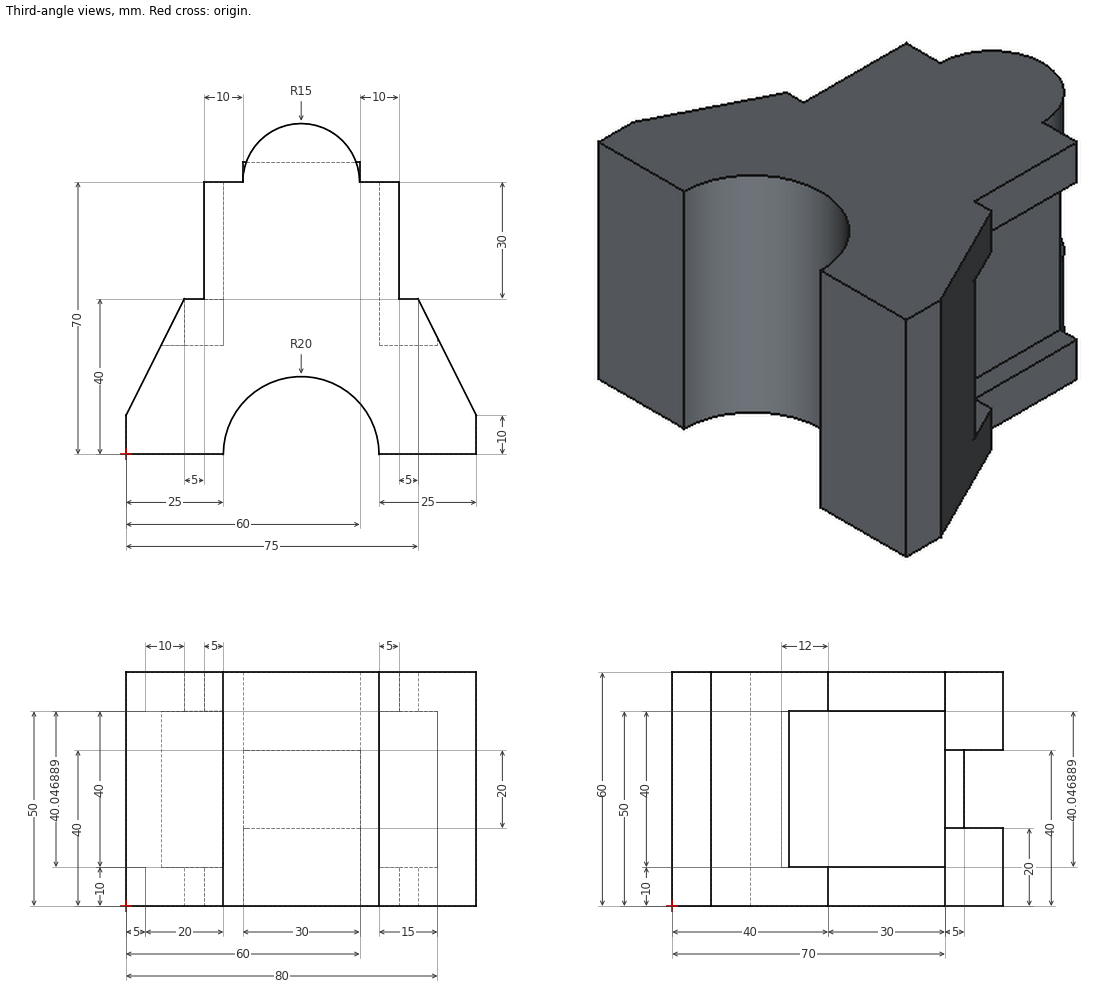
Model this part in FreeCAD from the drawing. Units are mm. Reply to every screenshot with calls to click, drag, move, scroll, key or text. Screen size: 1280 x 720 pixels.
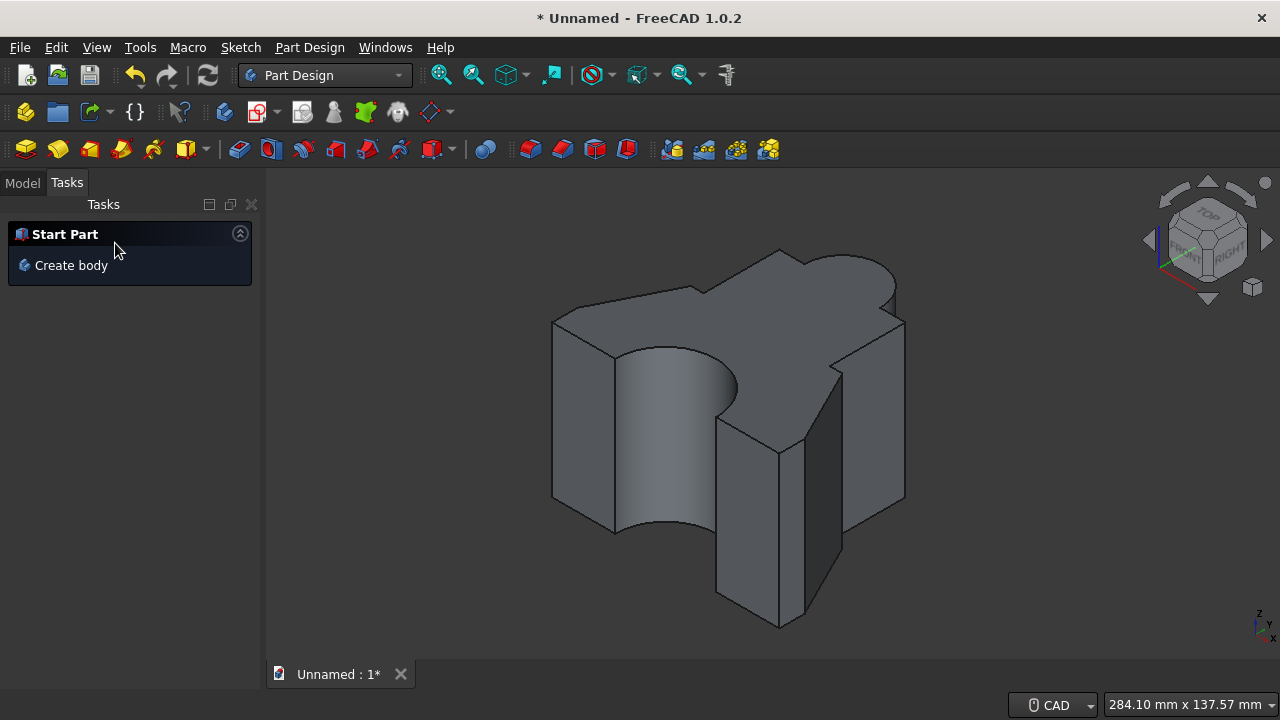
click(868, 406)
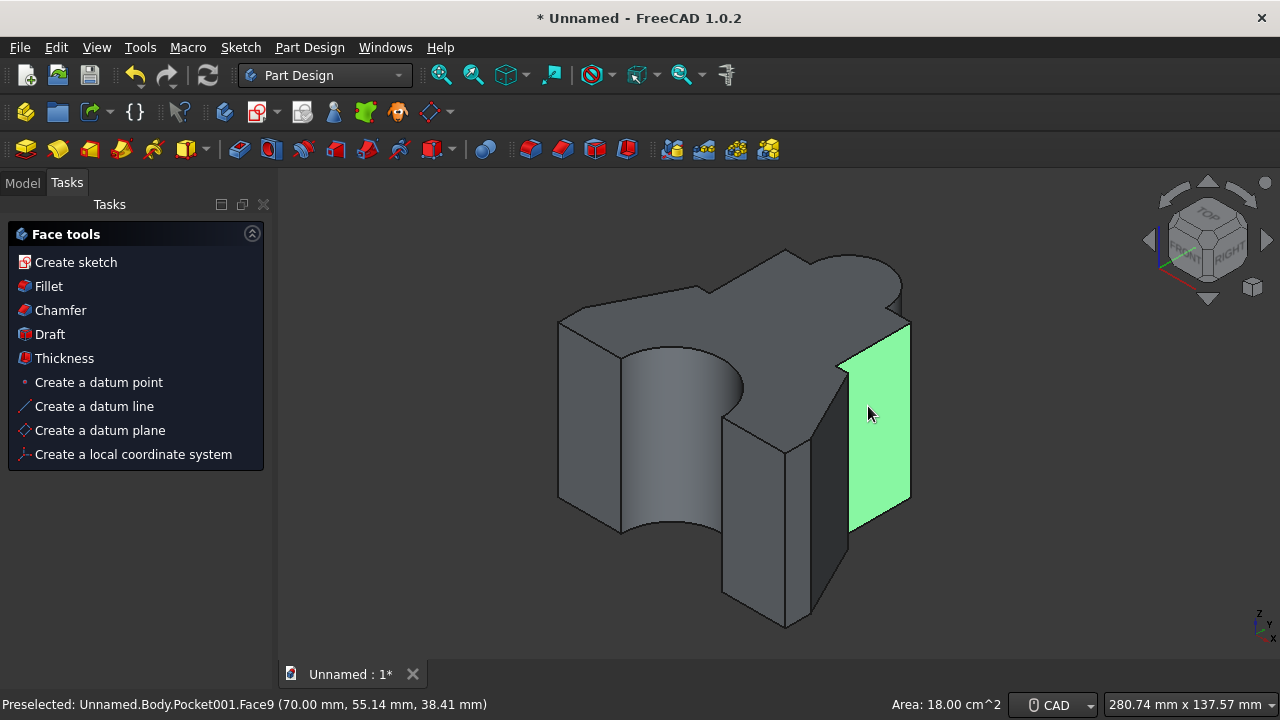
click(258, 112)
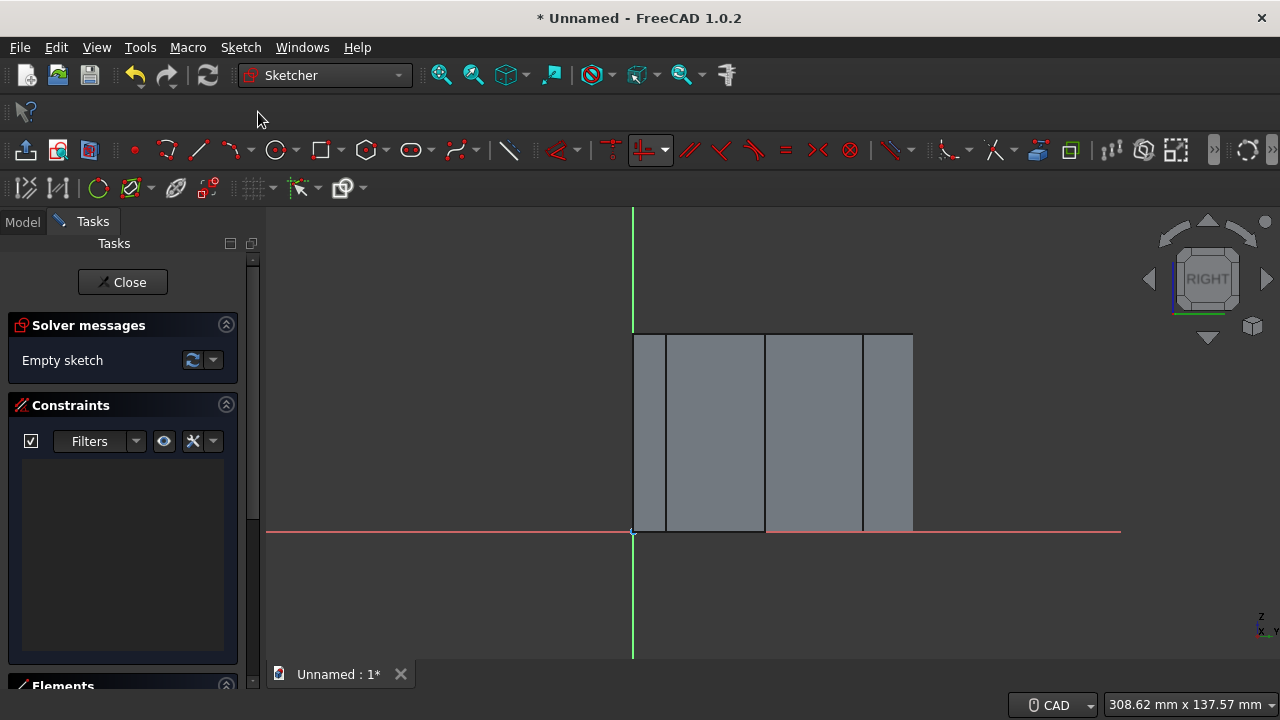
key(q)
key(s)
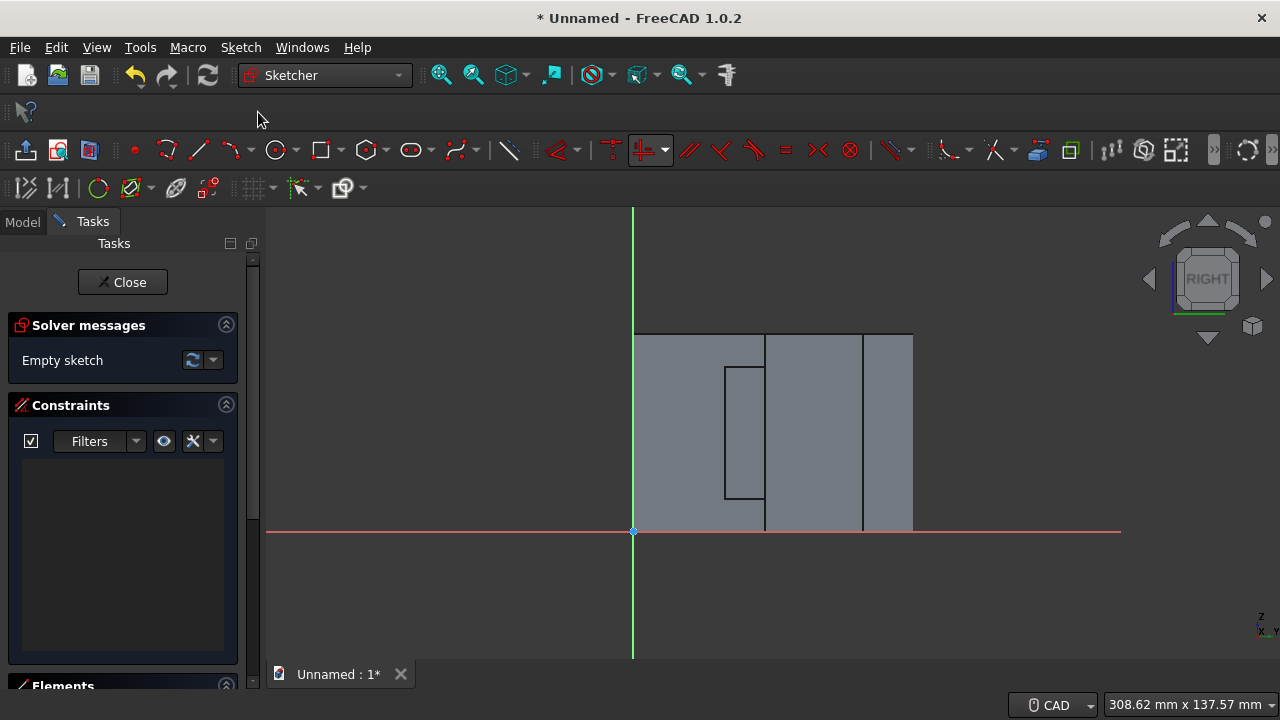
scroll(802, 469, up, 3)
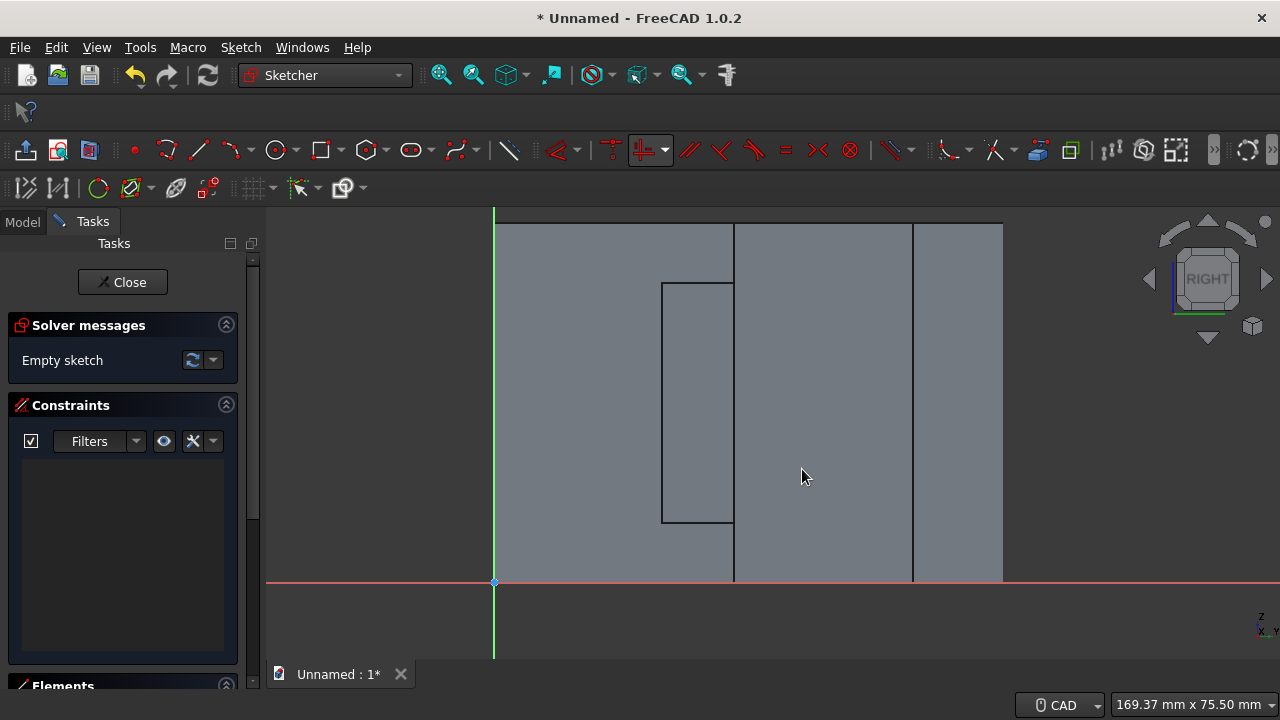
key(g)
key(r)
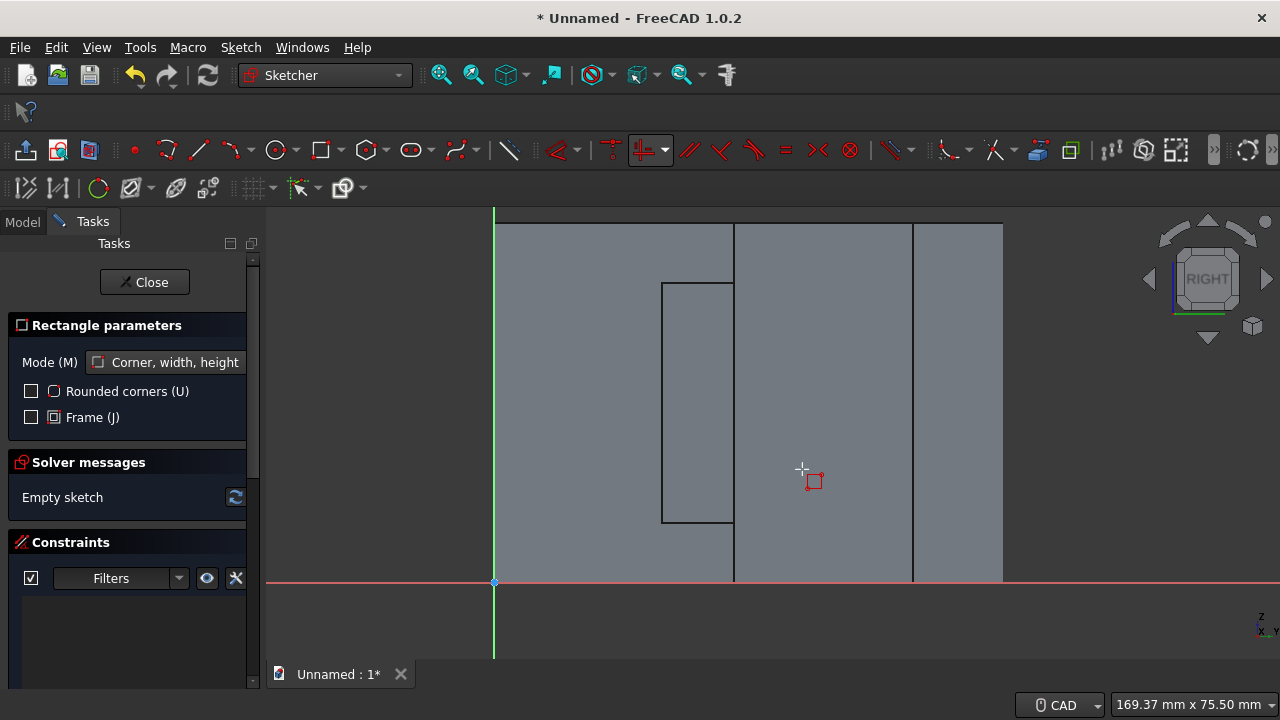
click(734, 283)
click(913, 523)
key(Escape)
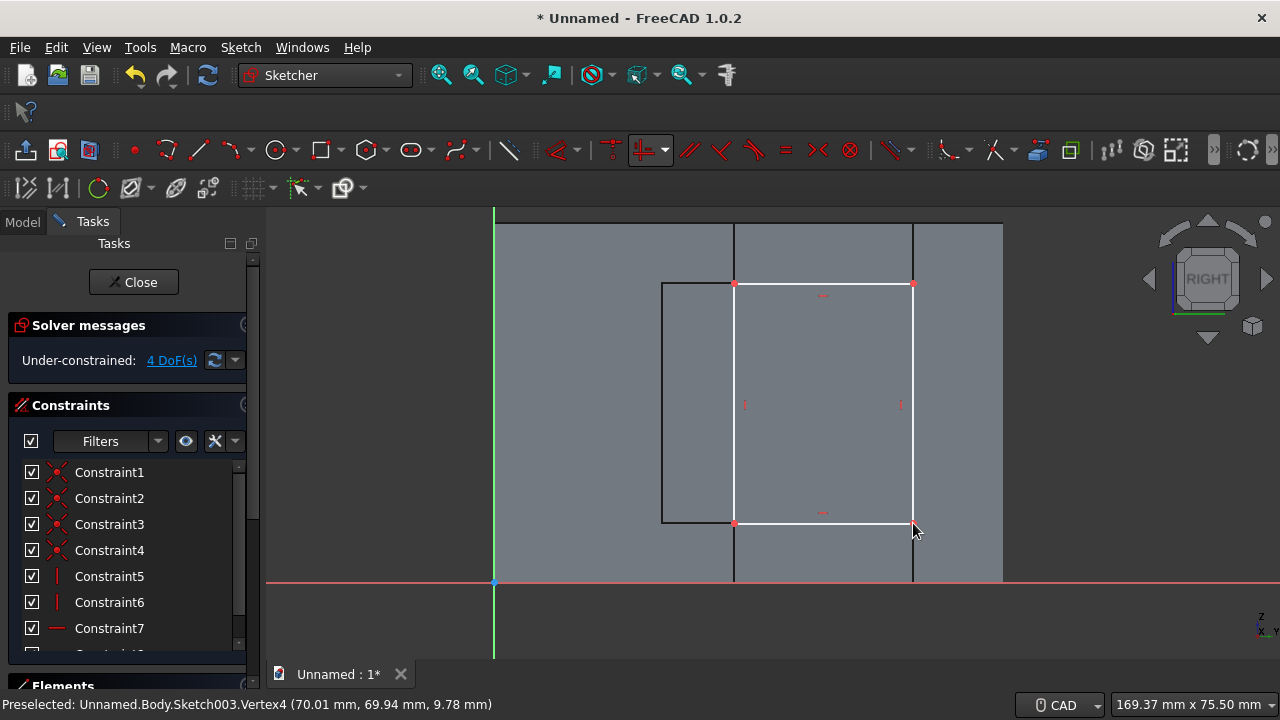
key(d)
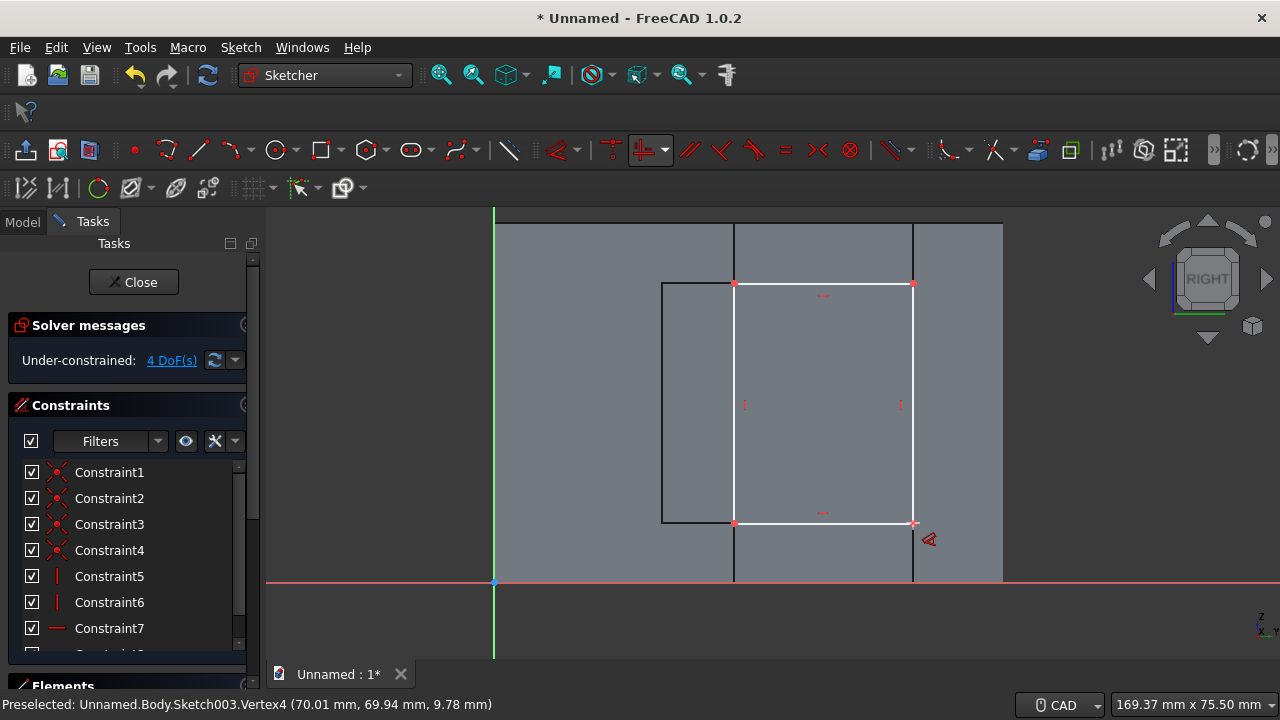
click(734, 356)
click(768, 404)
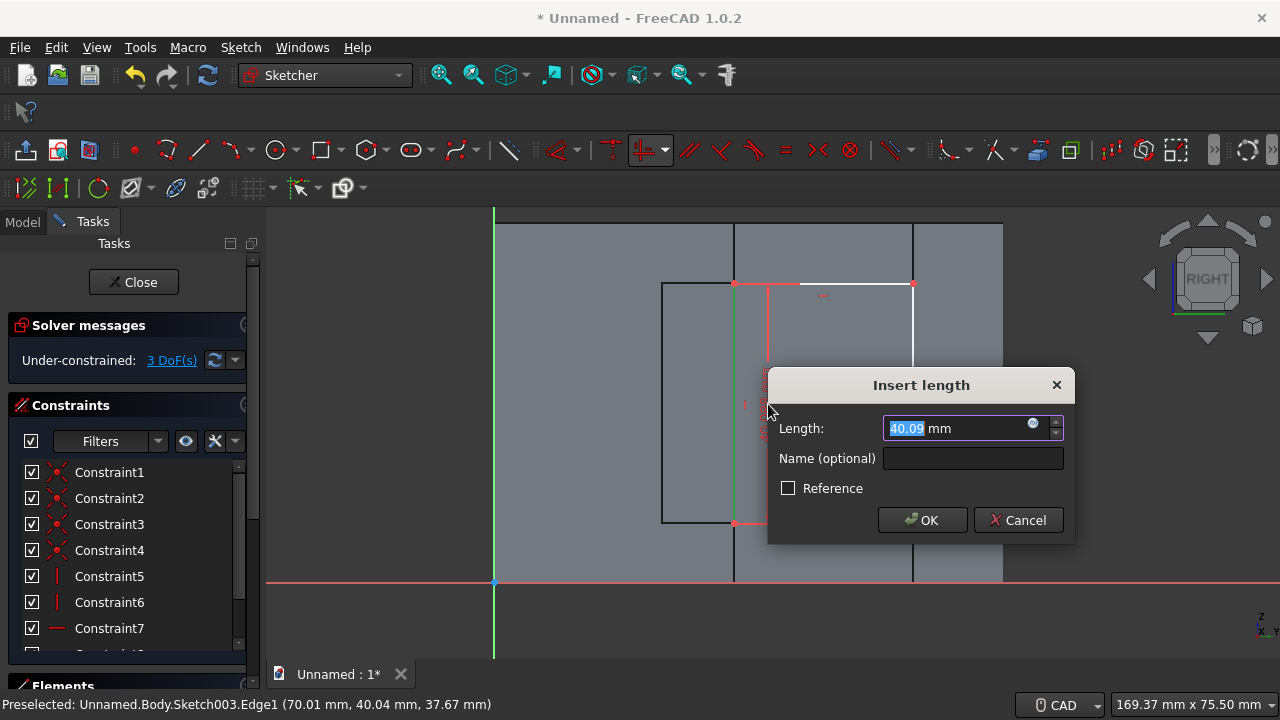
text(40)
key(Return)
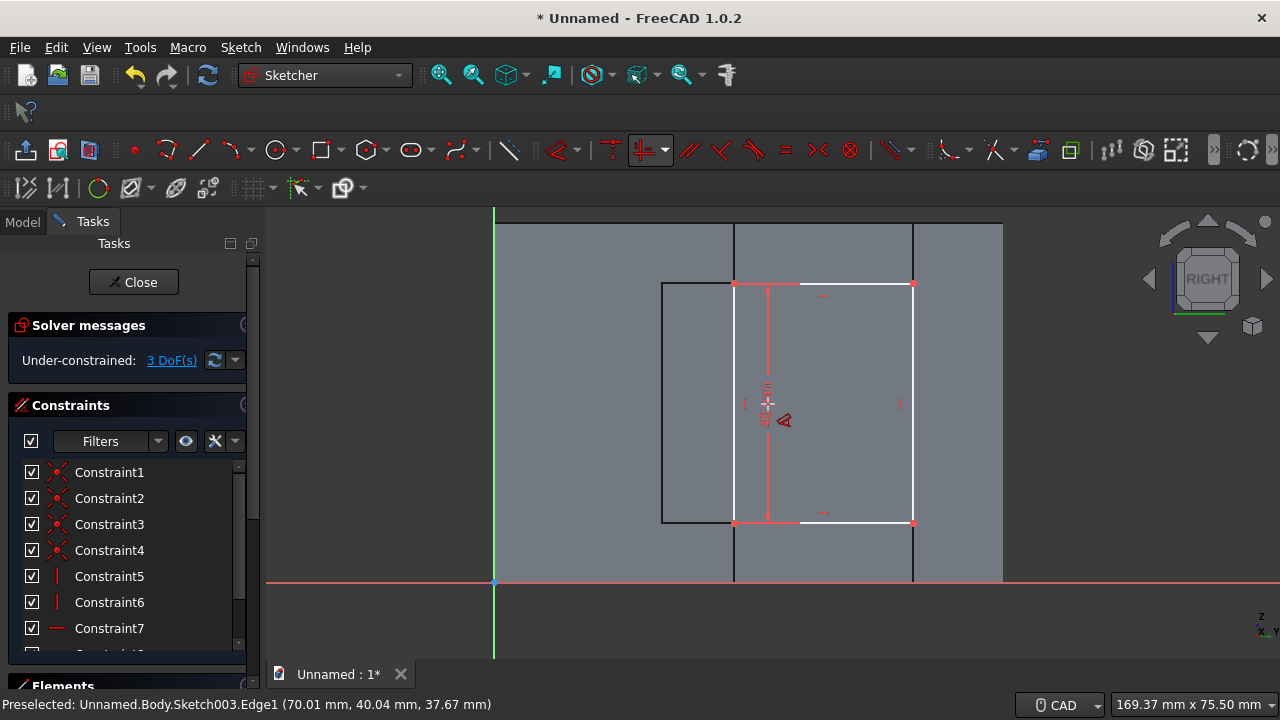
click(788, 523)
click(824, 557)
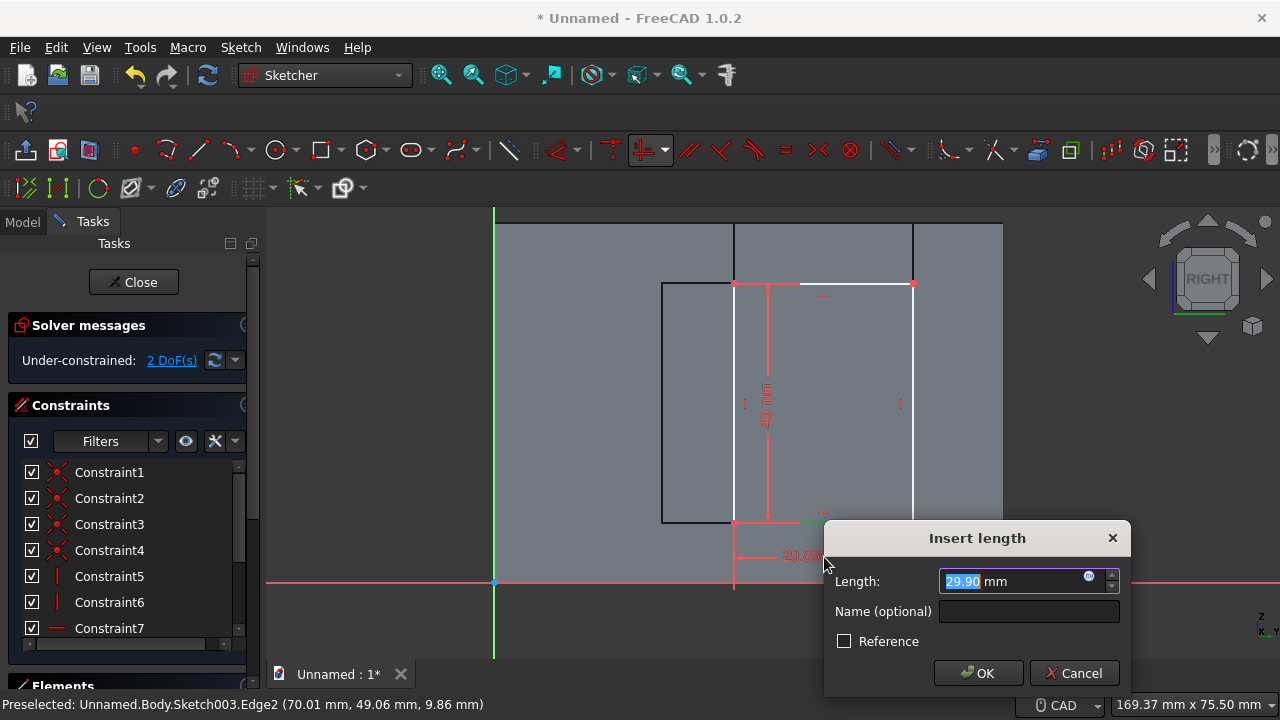
text(30)
key(Return)